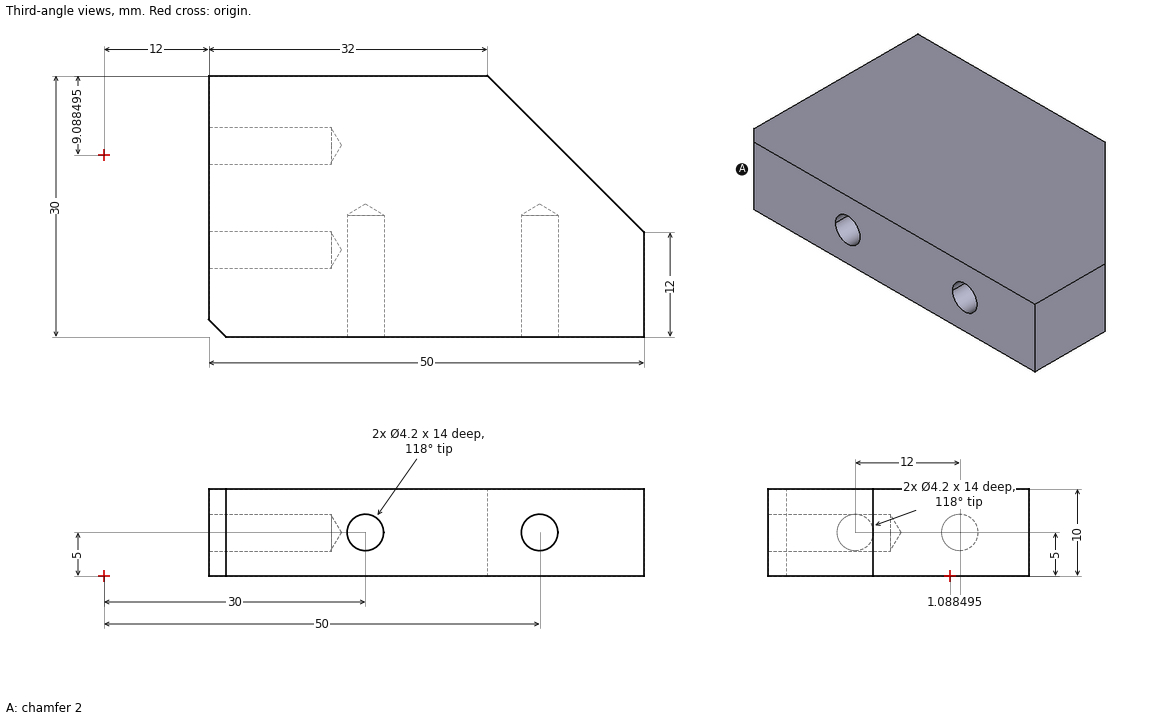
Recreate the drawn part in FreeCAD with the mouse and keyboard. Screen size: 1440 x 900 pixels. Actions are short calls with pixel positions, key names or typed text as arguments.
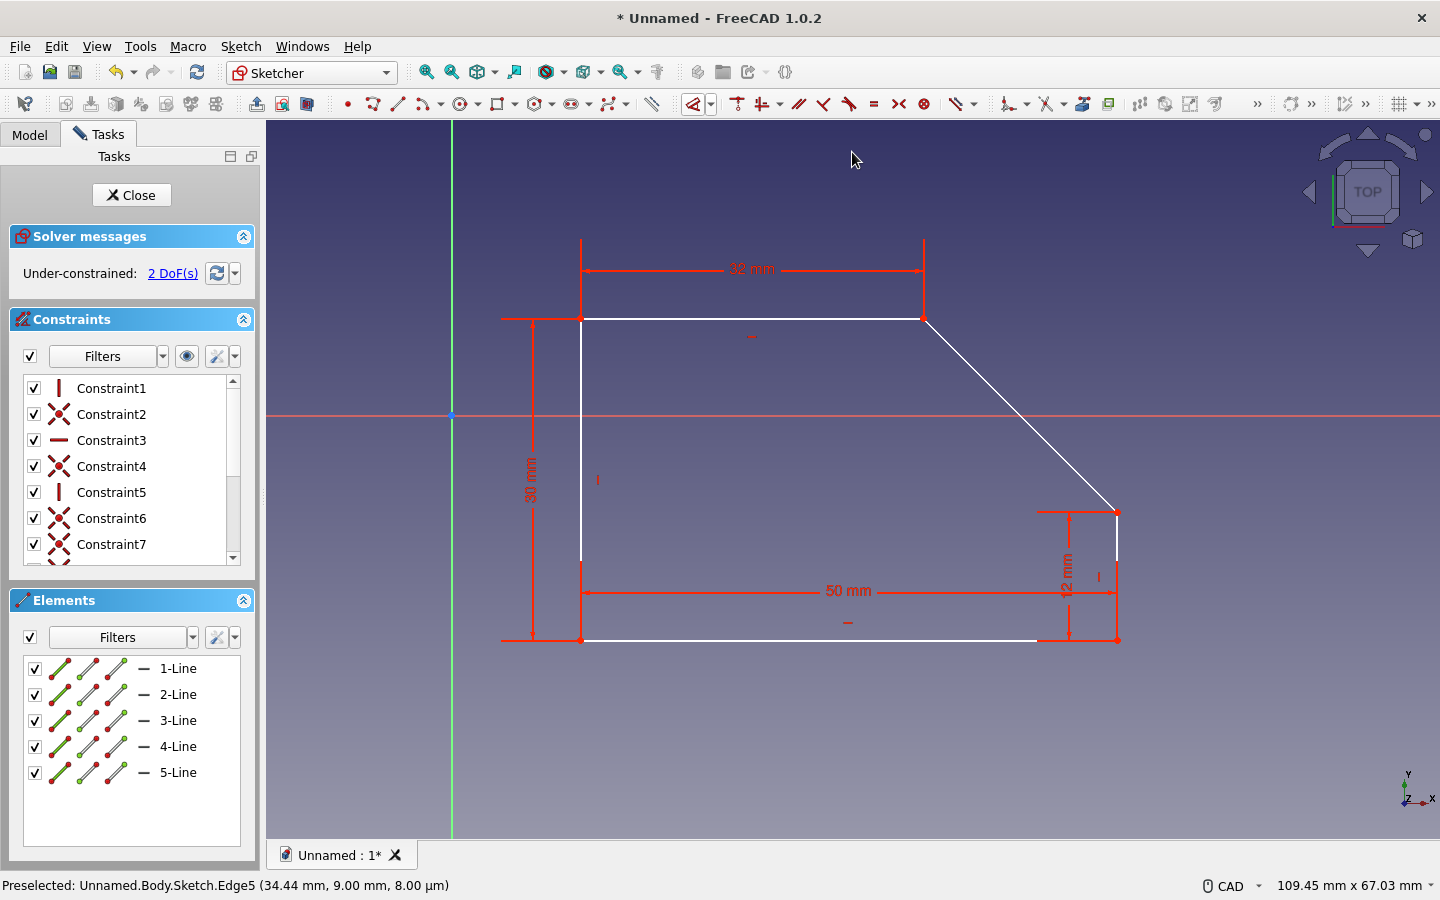
click(581, 319)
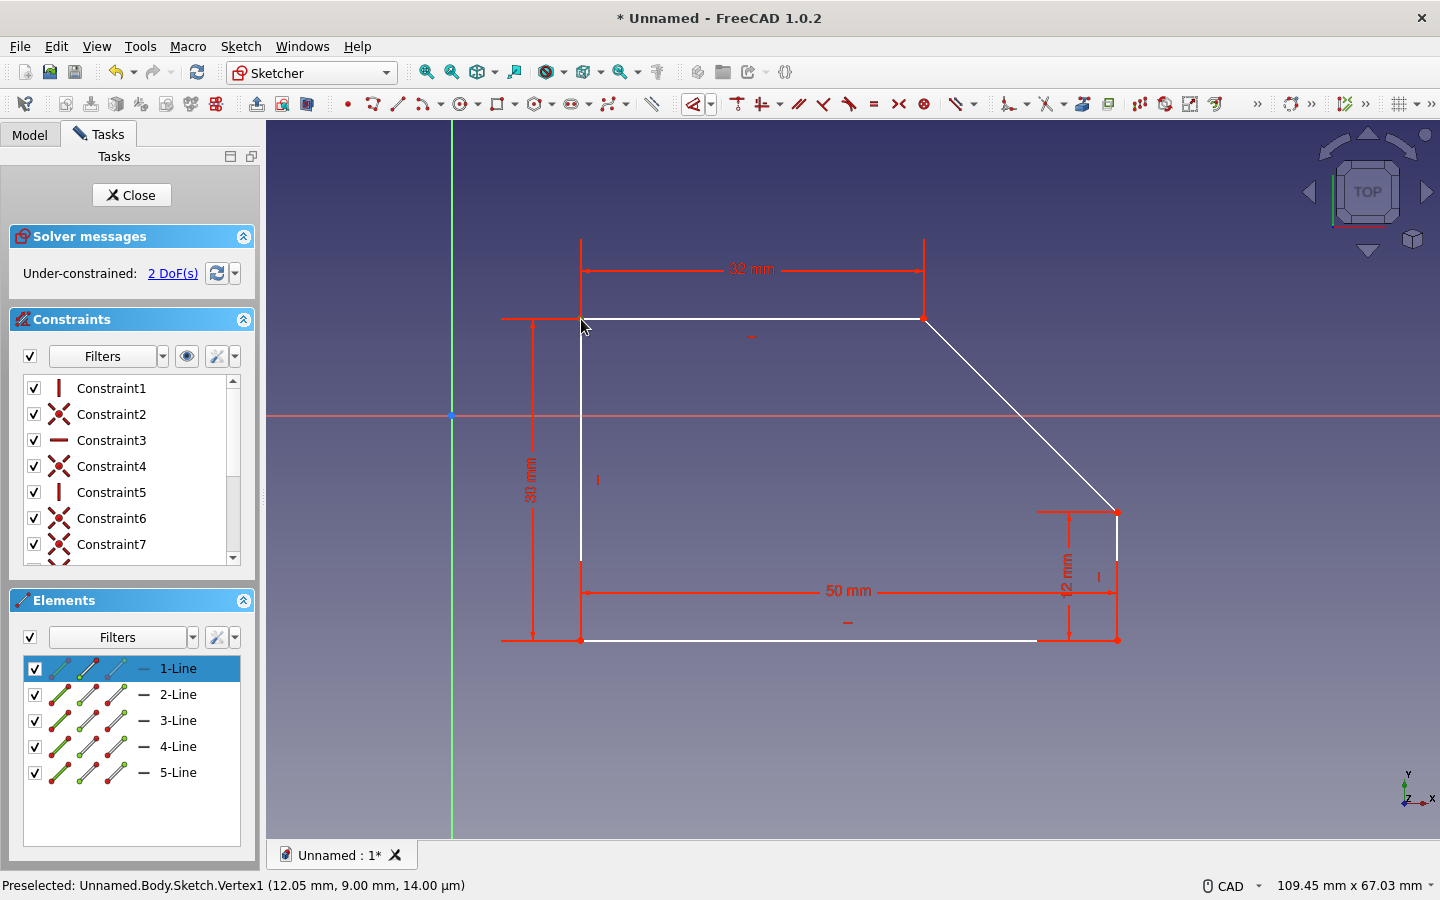
click(710, 104)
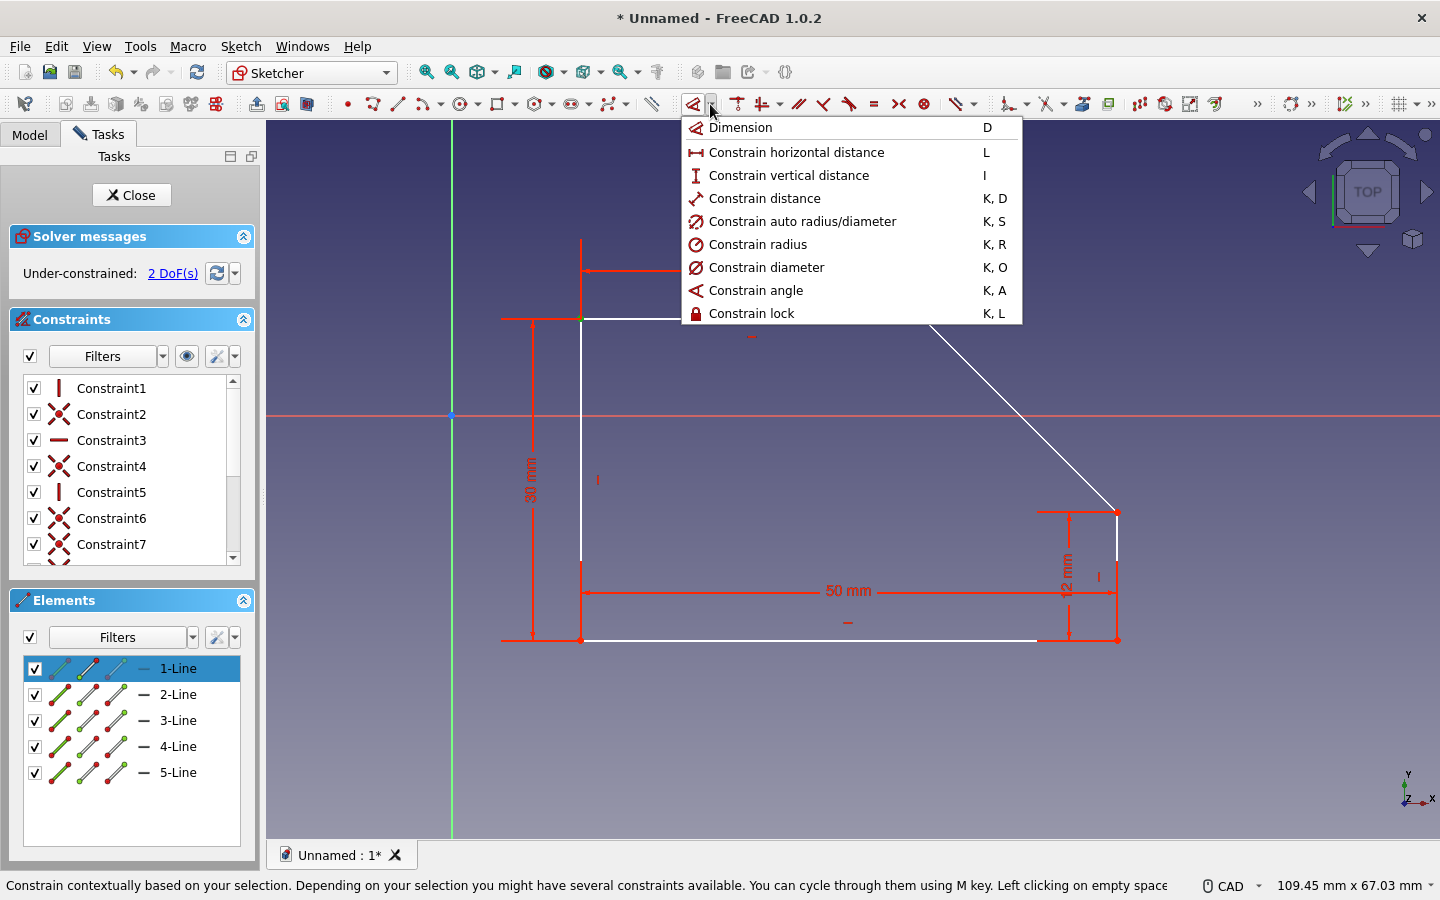
click(852, 152)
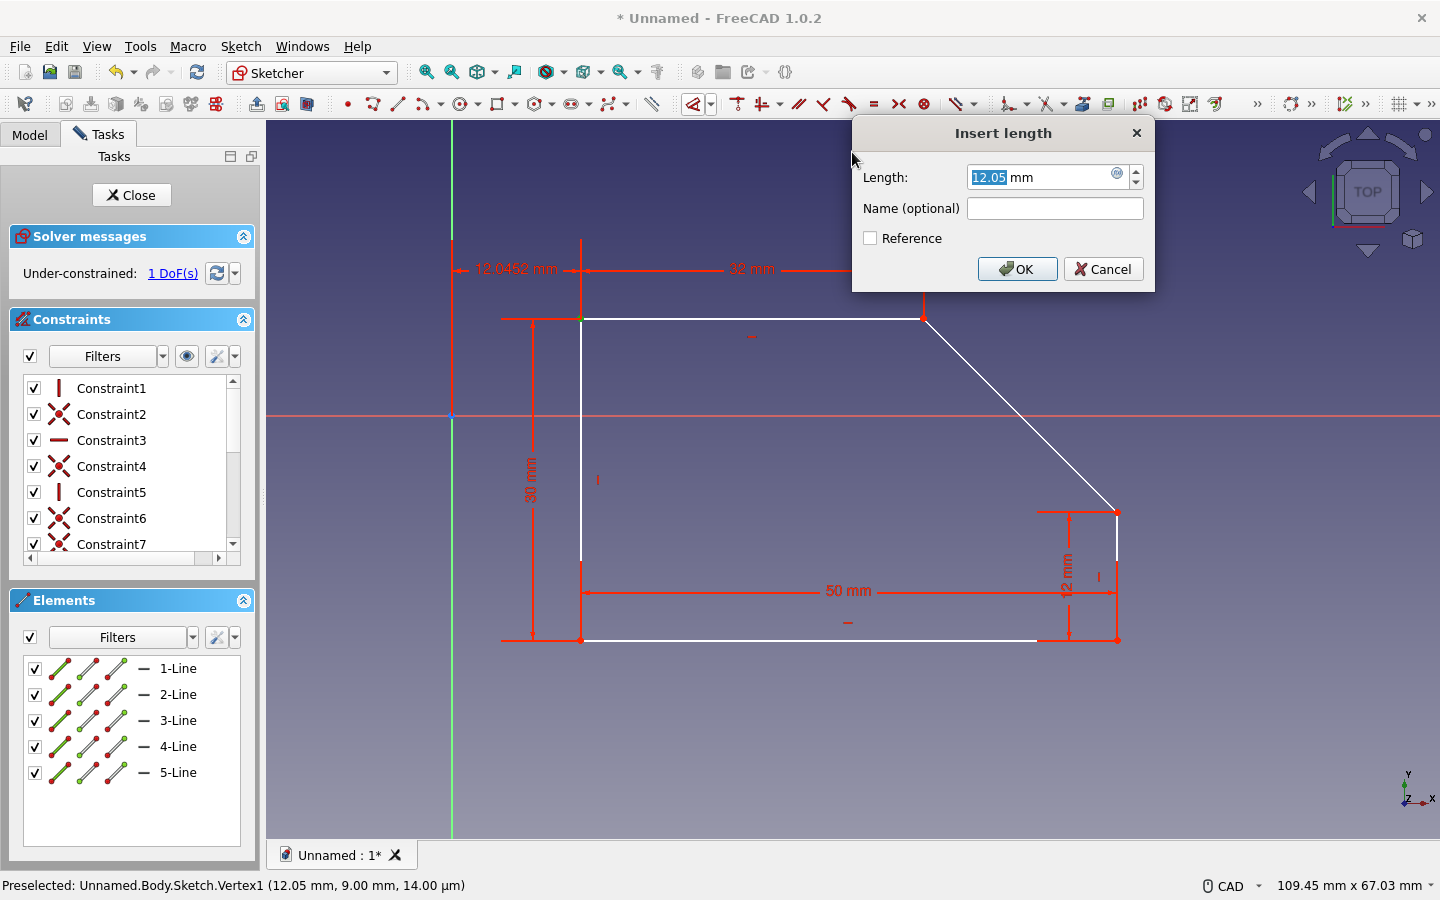
text(12)
key(Return)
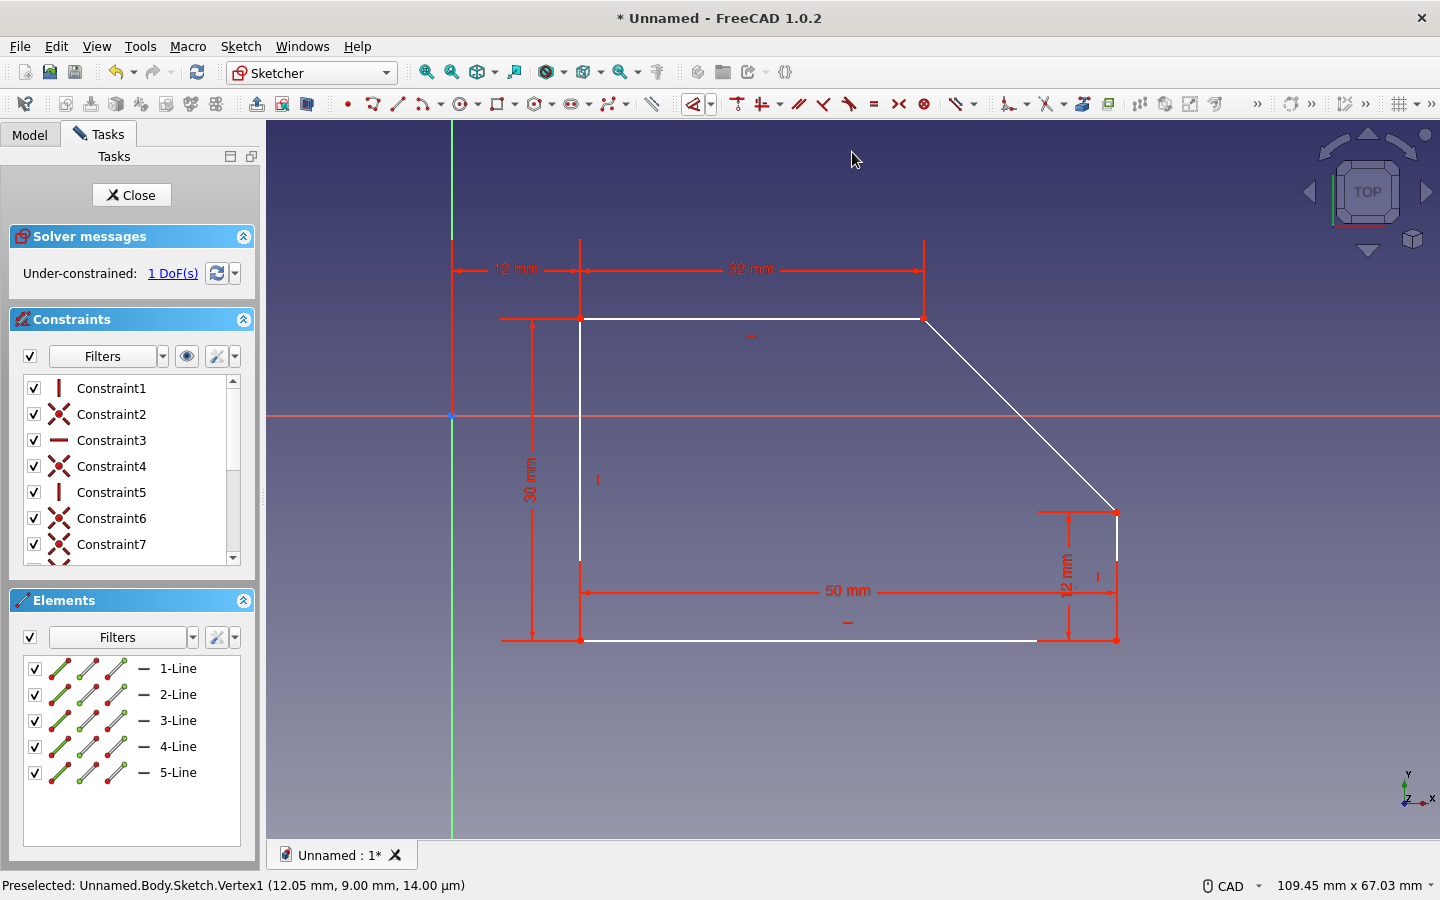
click(580, 319)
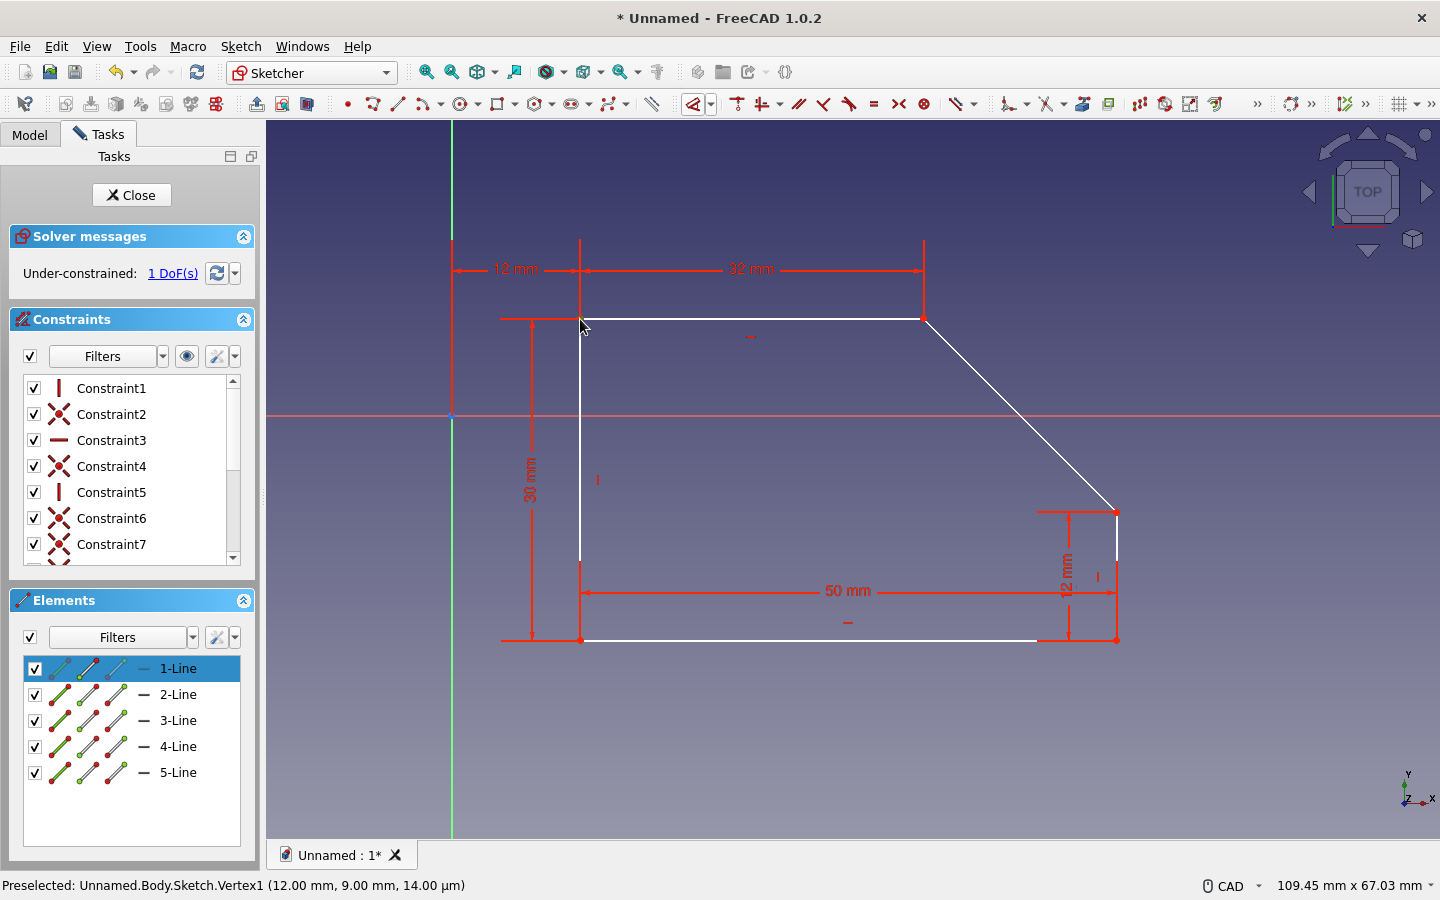
click(710, 104)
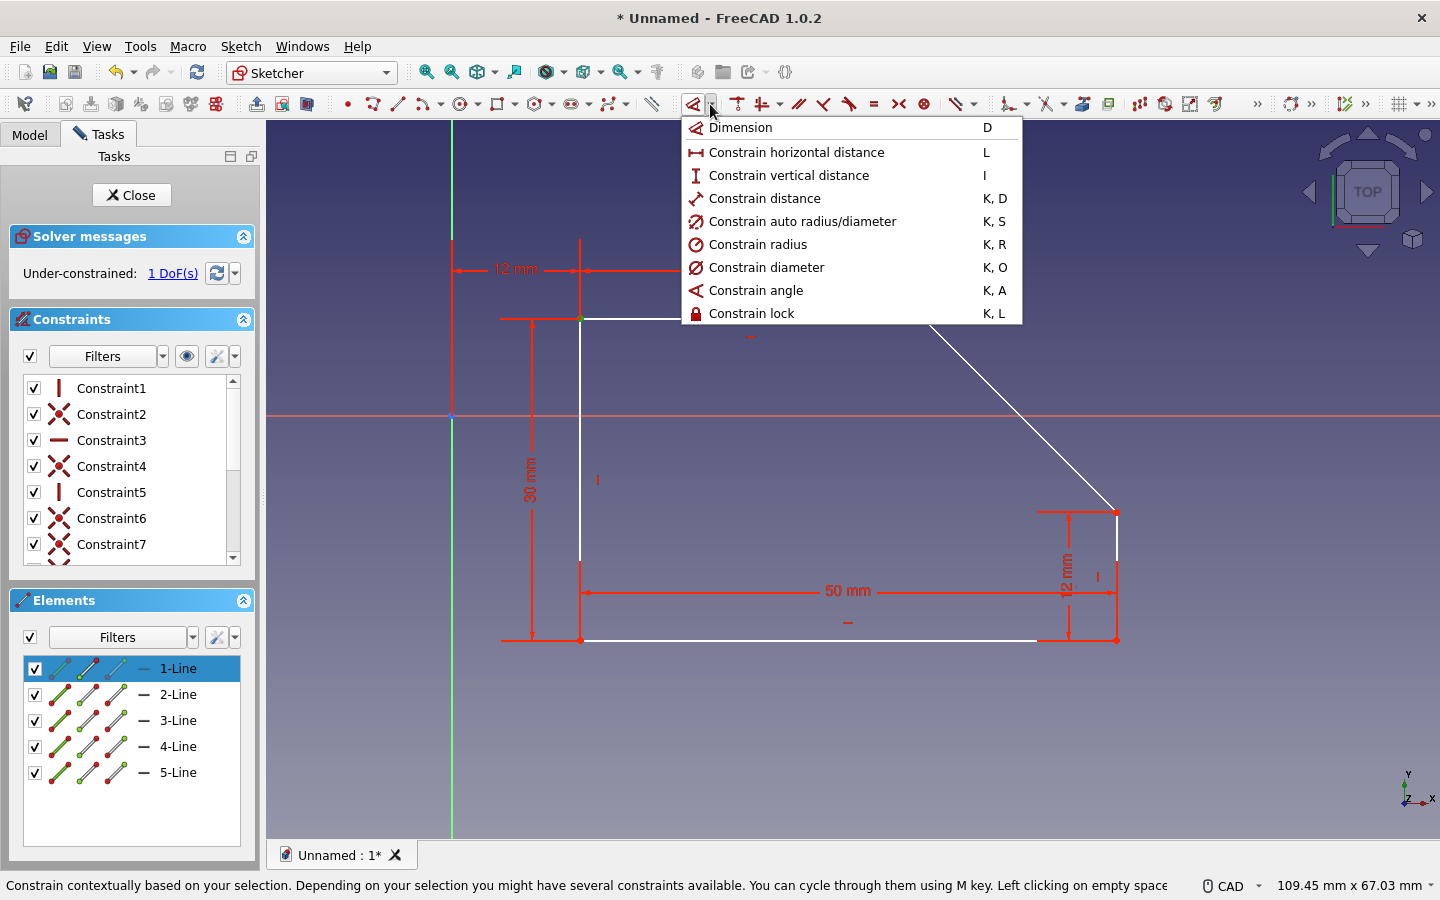
click(852, 176)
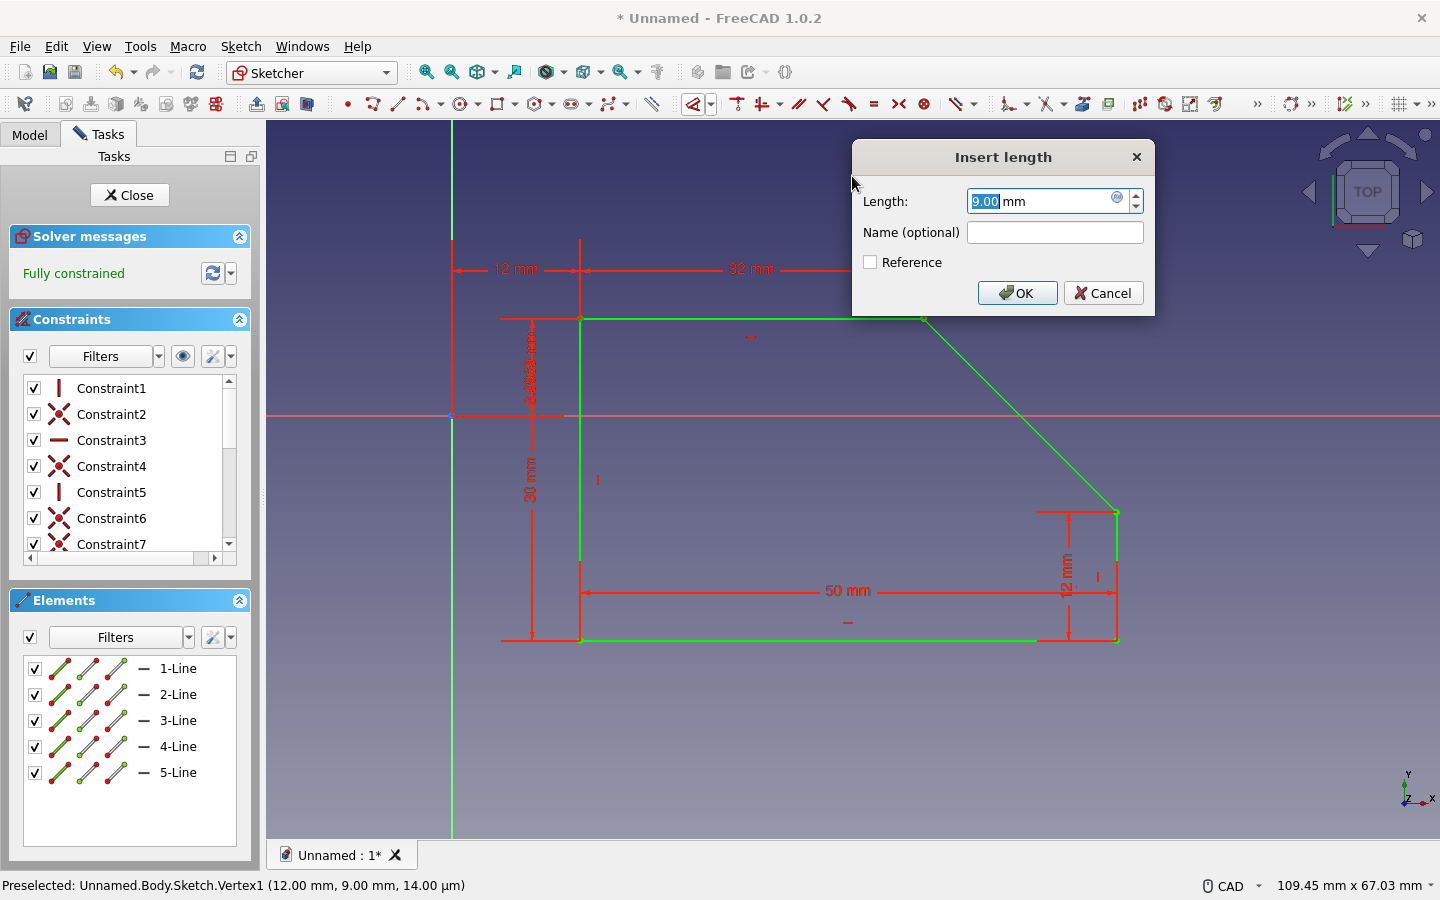
text(9.088495)
key(Return)